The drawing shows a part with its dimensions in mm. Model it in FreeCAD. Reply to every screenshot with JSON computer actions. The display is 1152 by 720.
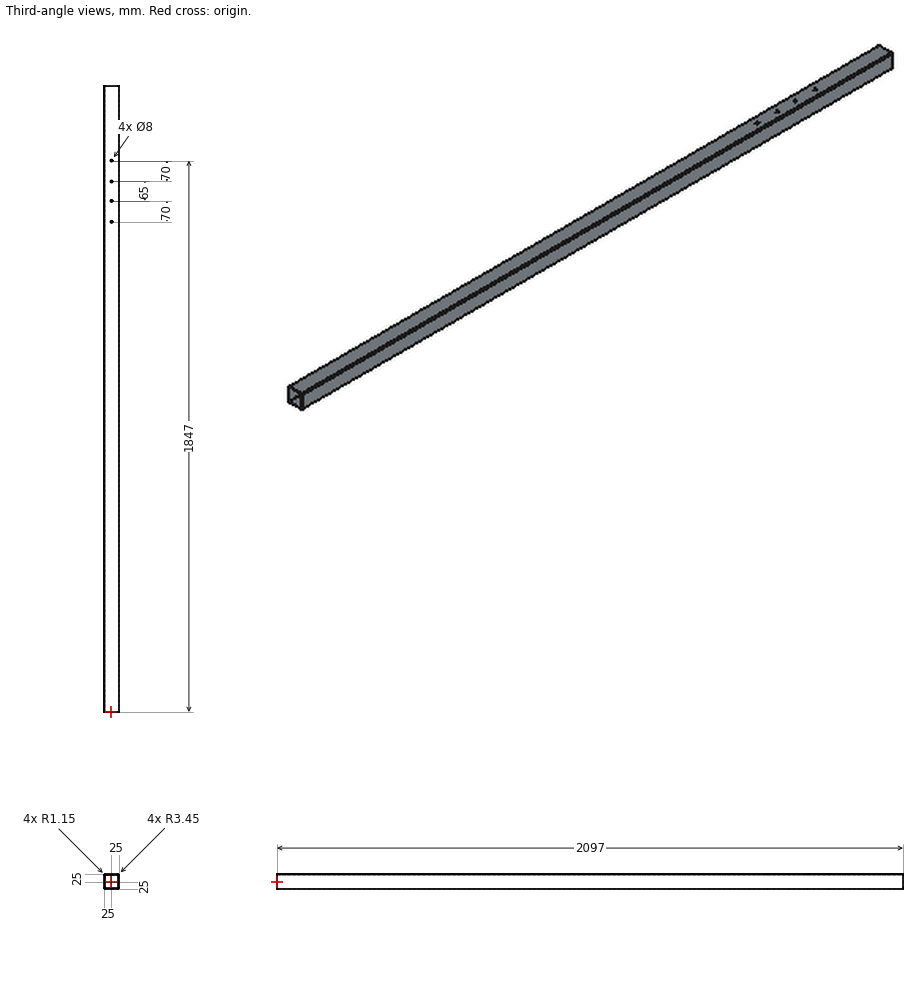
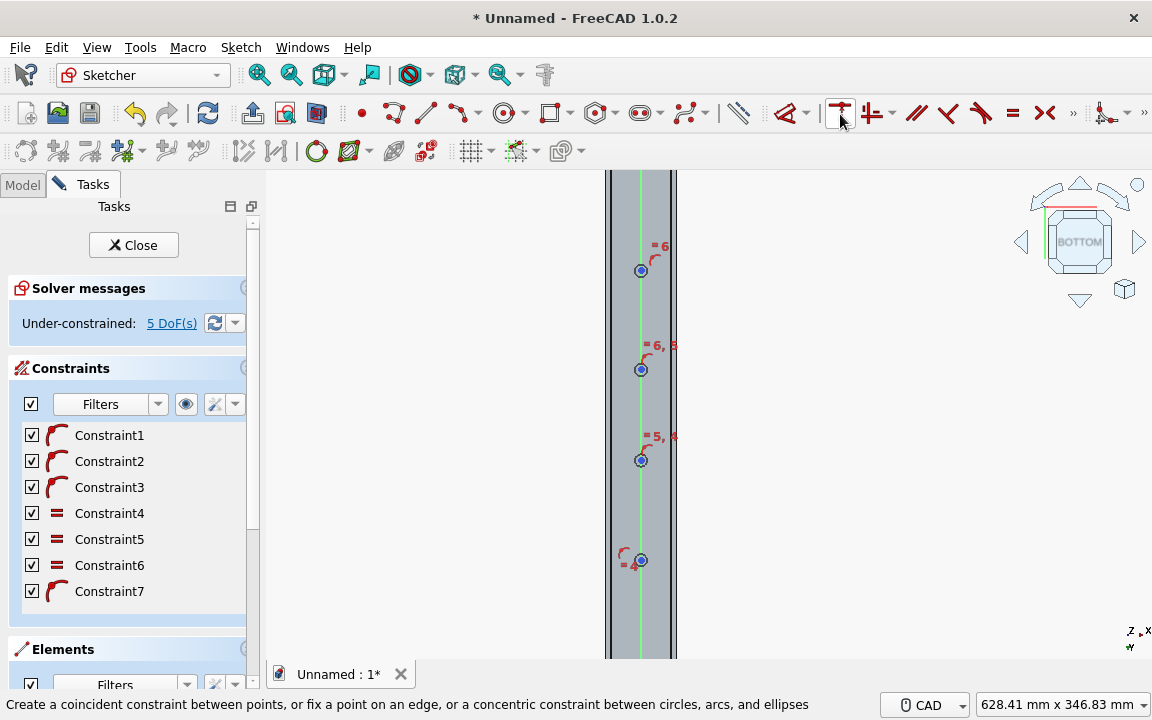
{"action": "left_click", "coordinate": [786, 114]}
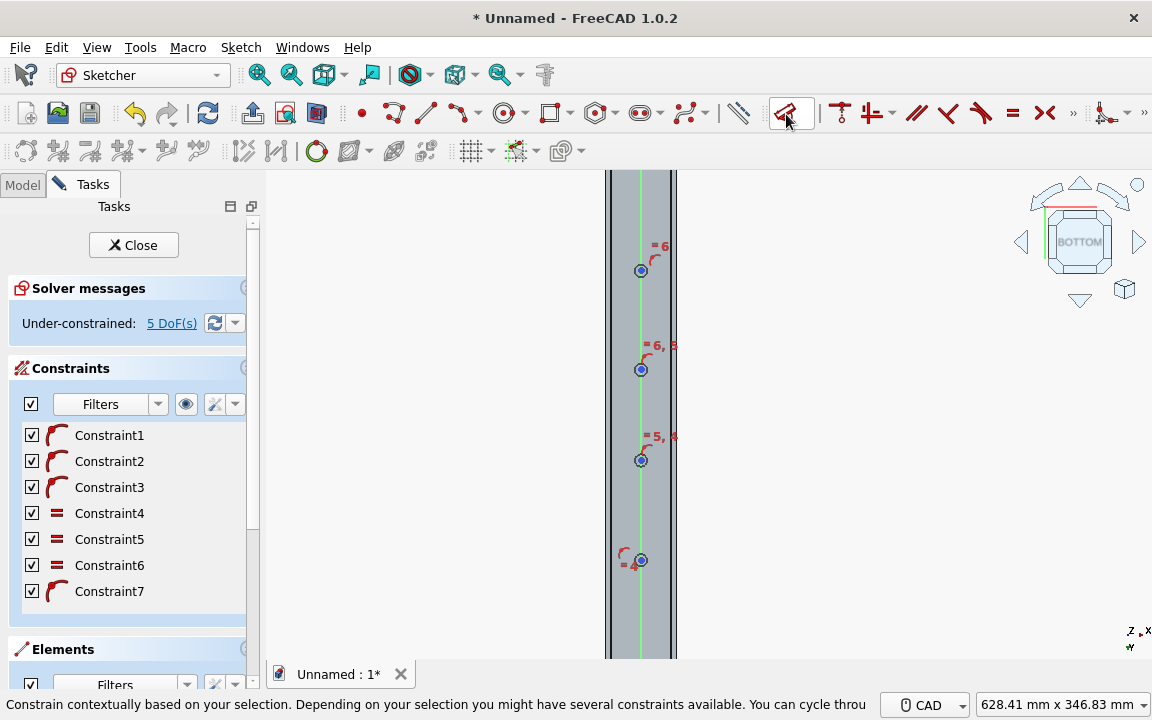
{"action": "scroll", "coordinate": [641, 554], "scroll_direction": "up", "scroll_amount": 7}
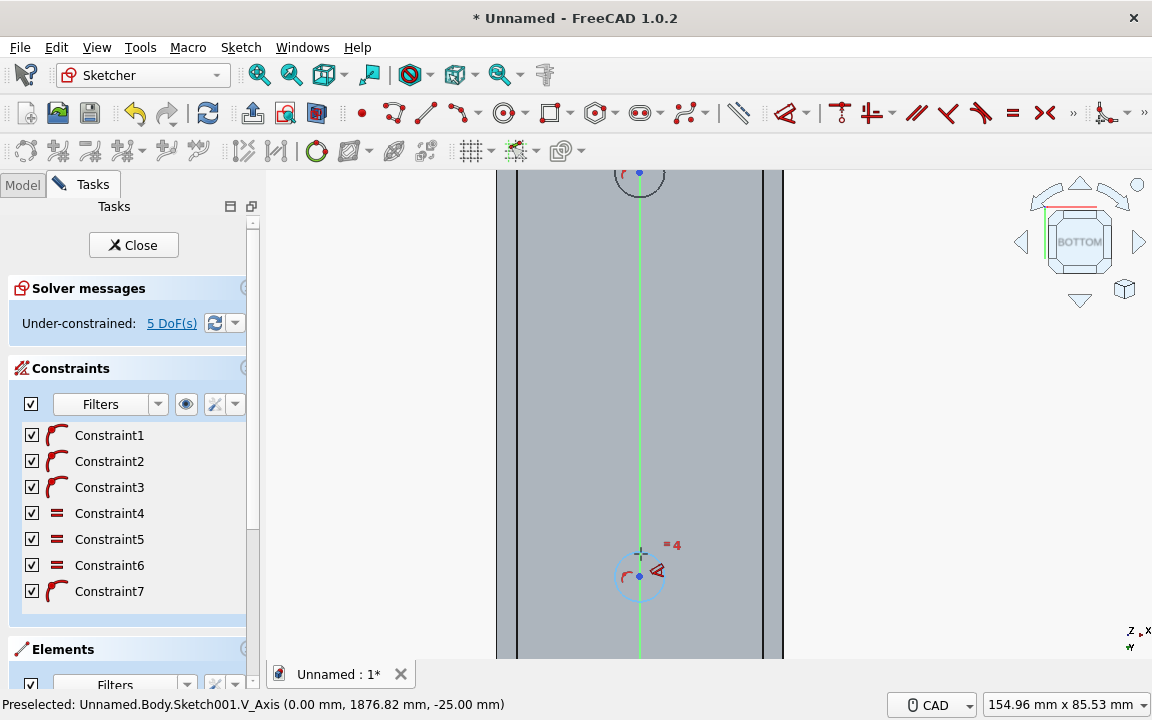
{"action": "left_click", "coordinate": [640, 552]}
{"action": "left_click", "coordinate": [668, 527]}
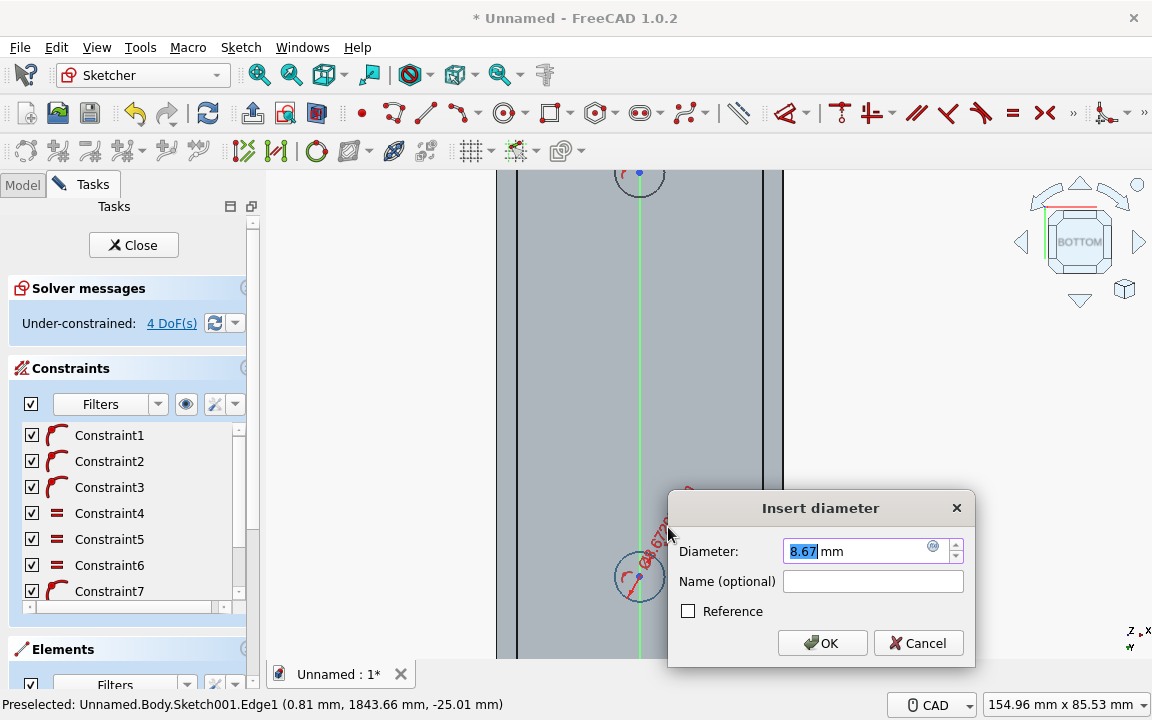
{"action": "type", "text": "8"}
{"action": "key", "text": "Return"}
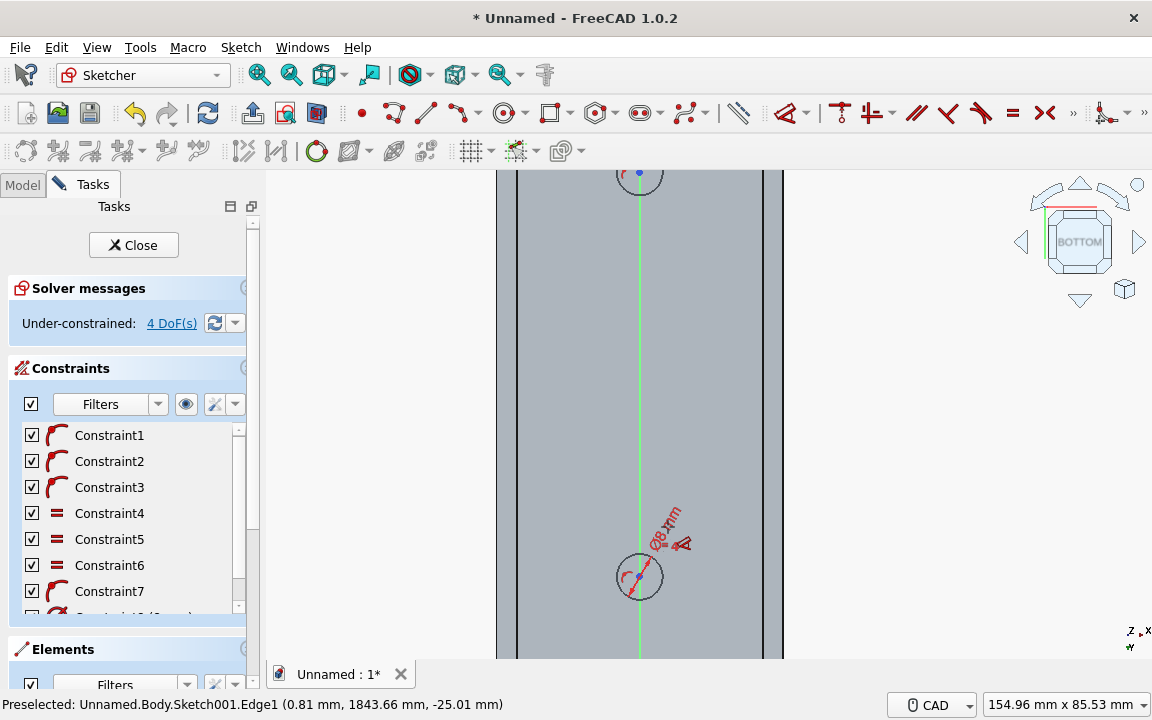
{"action": "scroll", "coordinate": [641, 555], "scroll_direction": "down", "scroll_amount": 7}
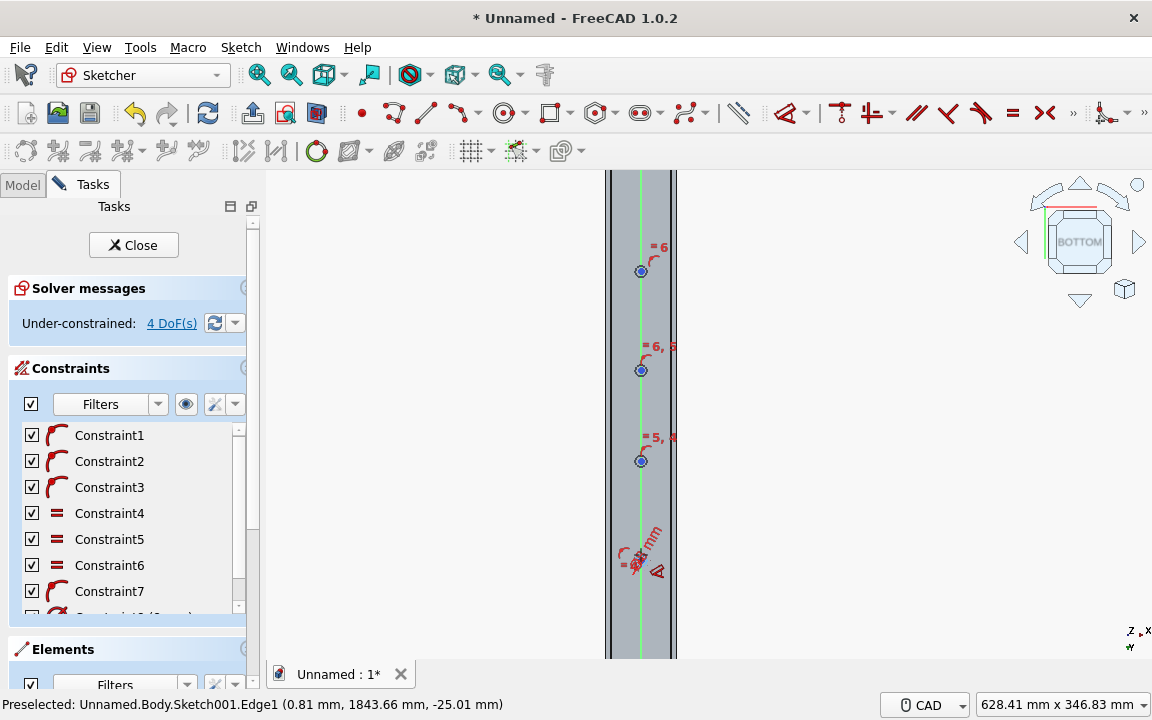
{"action": "left_click", "coordinate": [641, 561]}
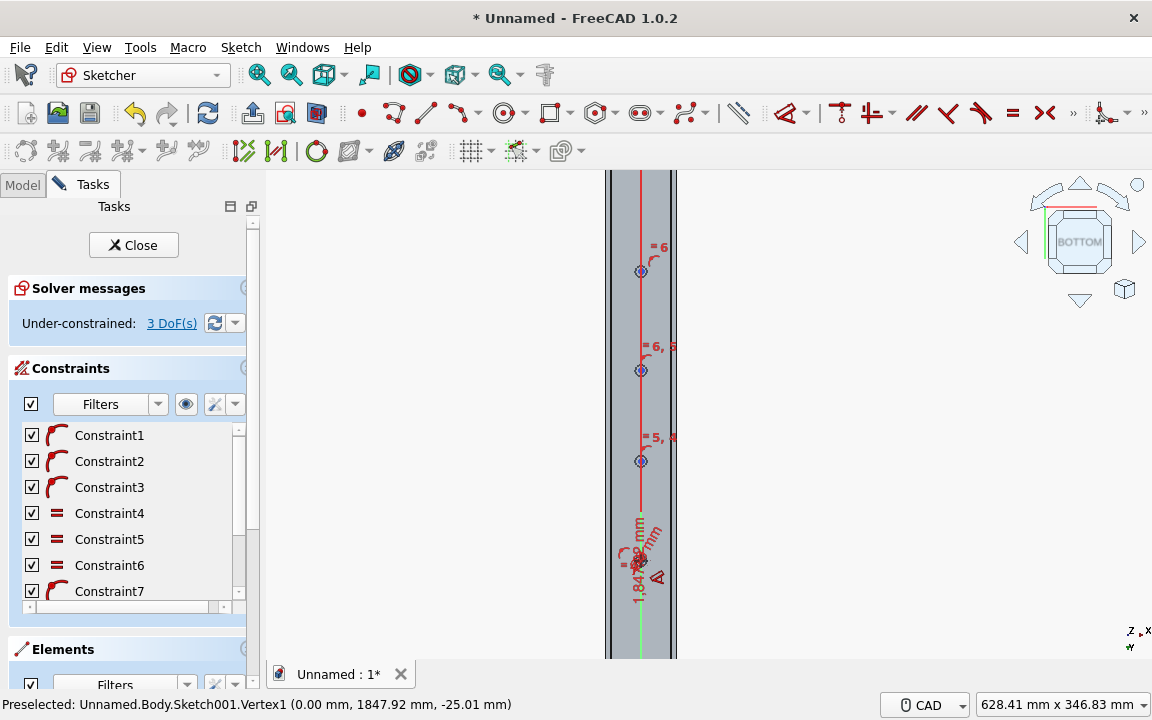
{"action": "left_click", "coordinate": [641, 461]}
{"action": "left_click", "coordinate": [675, 511]}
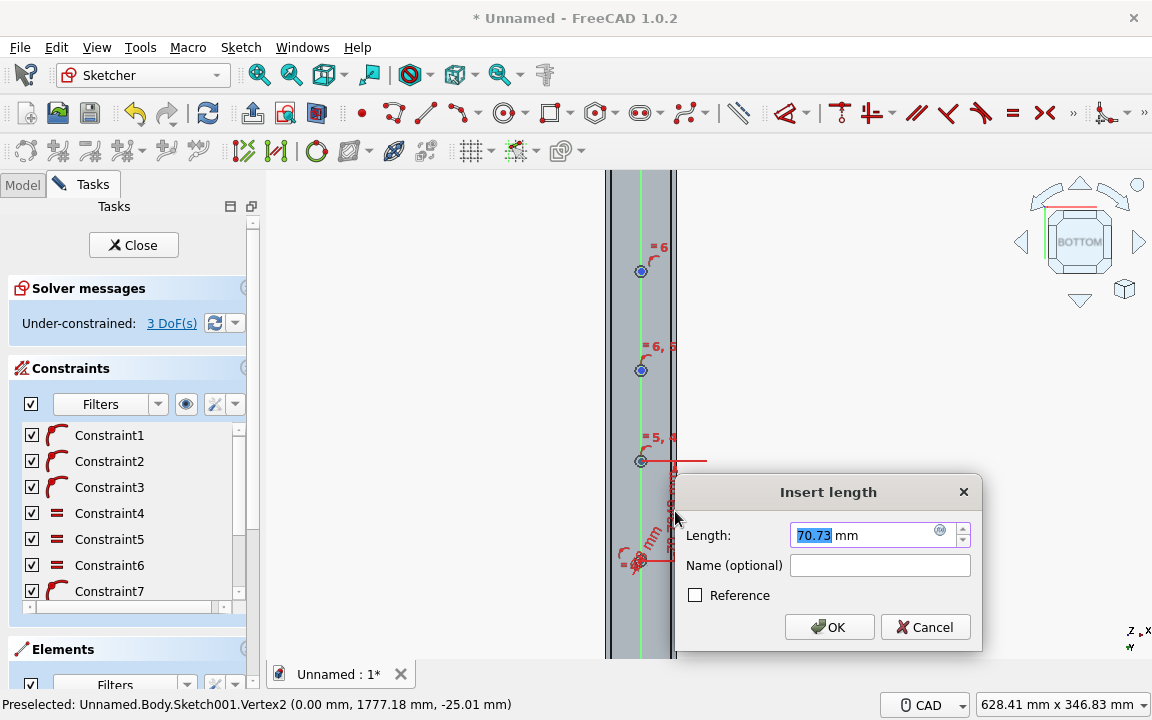
{"action": "type", "text": "70"}
{"action": "key", "text": "Return"}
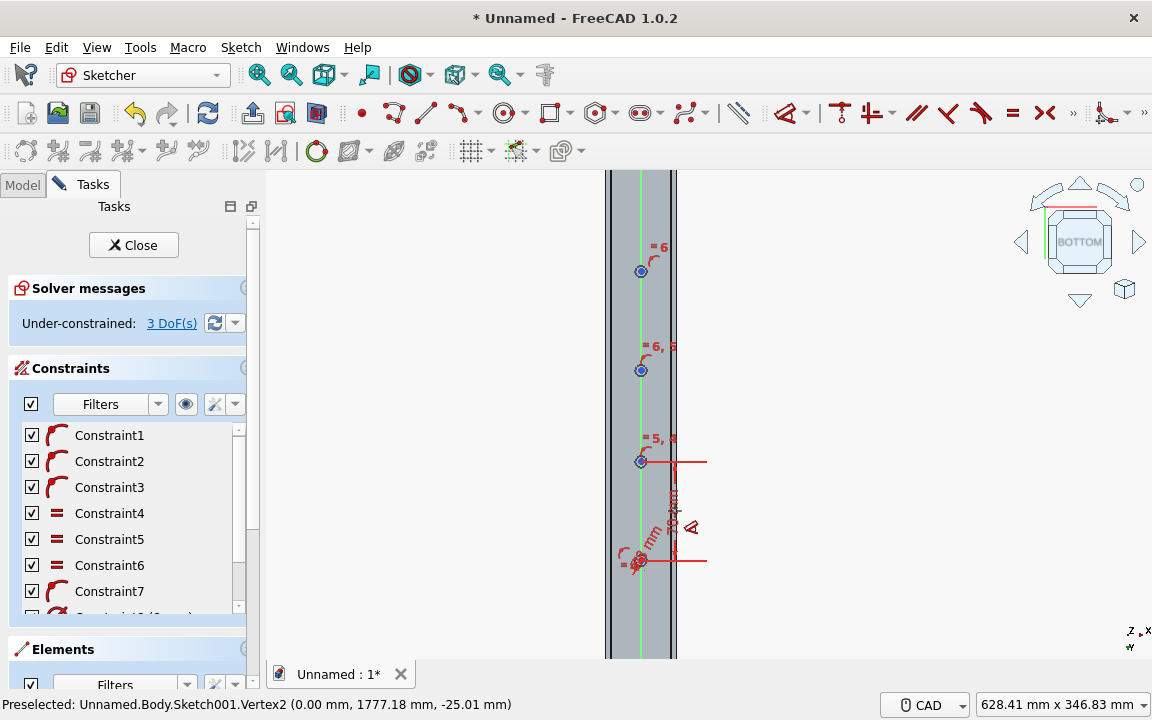
{"action": "left_click", "coordinate": [641, 462]}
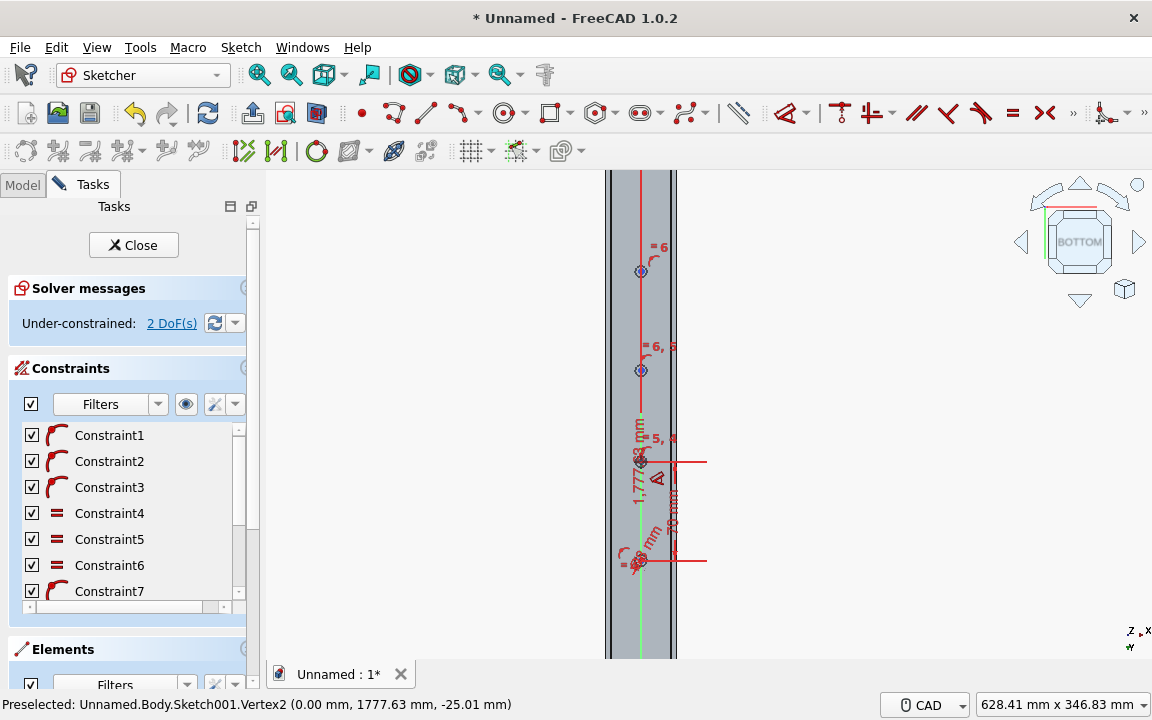
{"action": "left_click", "coordinate": [641, 371]}
{"action": "left_click", "coordinate": [675, 416]}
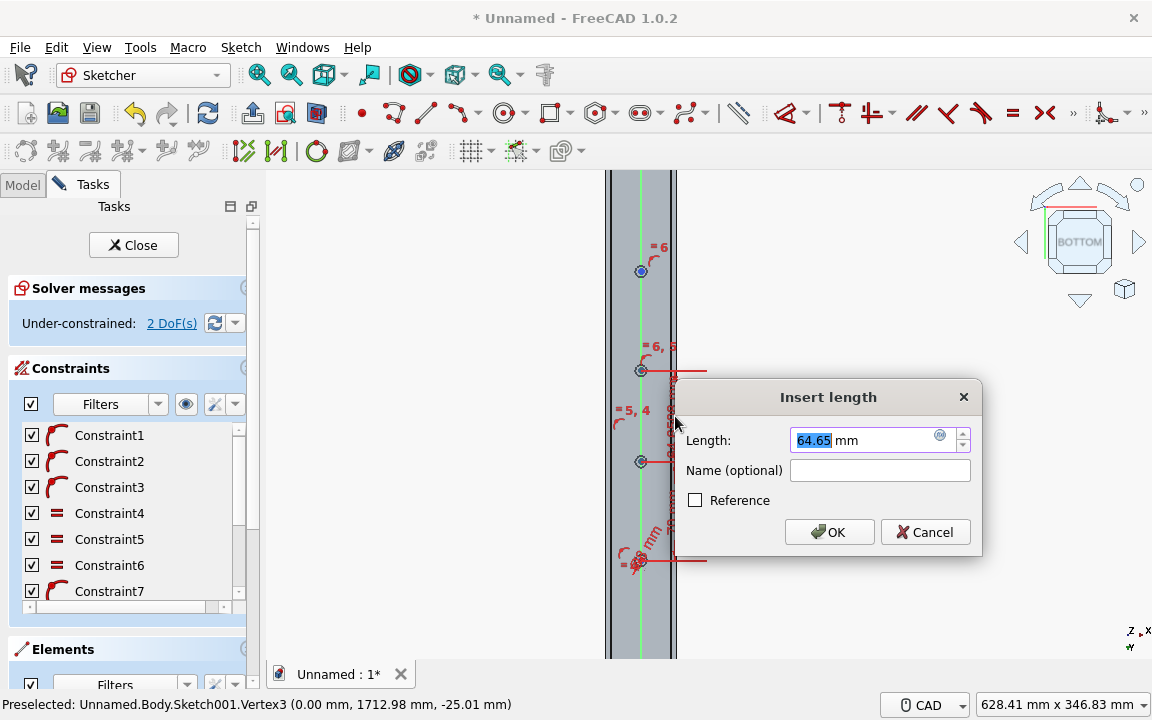
{"action": "type", "text": "65"}
{"action": "key", "text": "Return"}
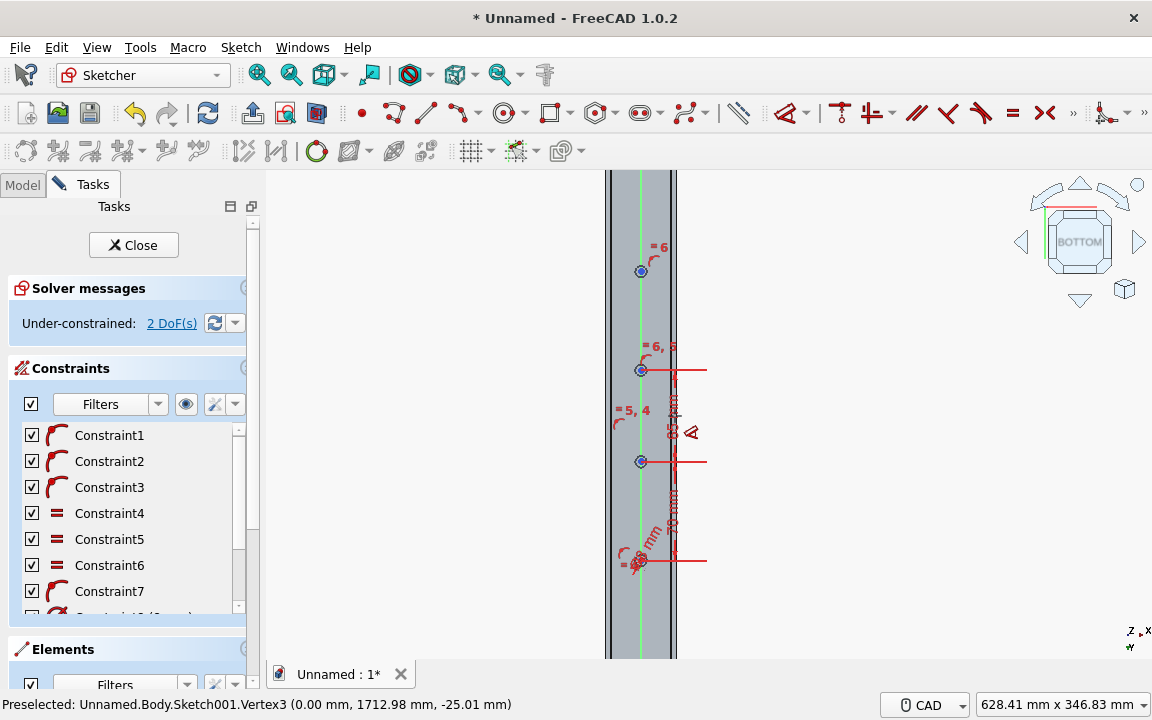
{"action": "left_click", "coordinate": [641, 370]}